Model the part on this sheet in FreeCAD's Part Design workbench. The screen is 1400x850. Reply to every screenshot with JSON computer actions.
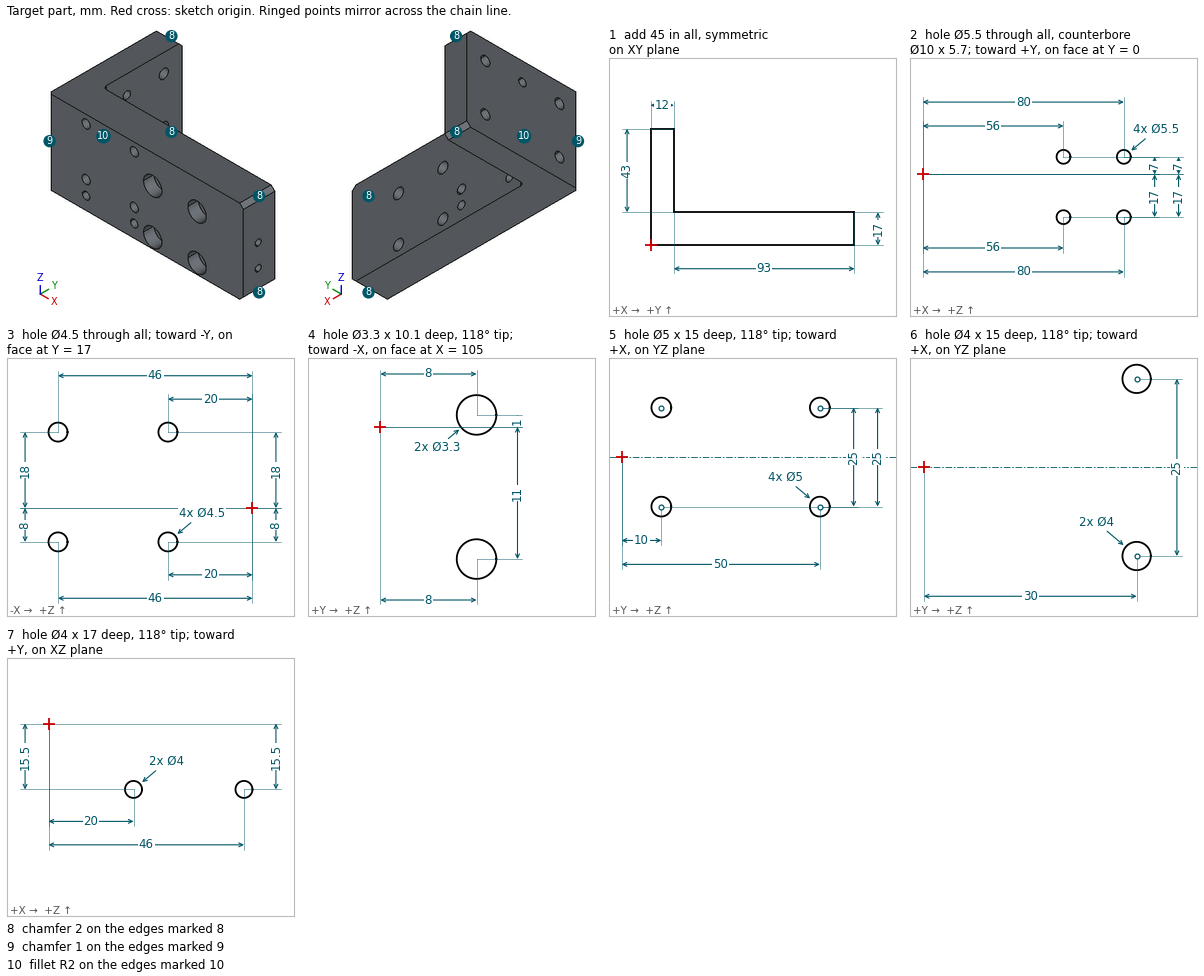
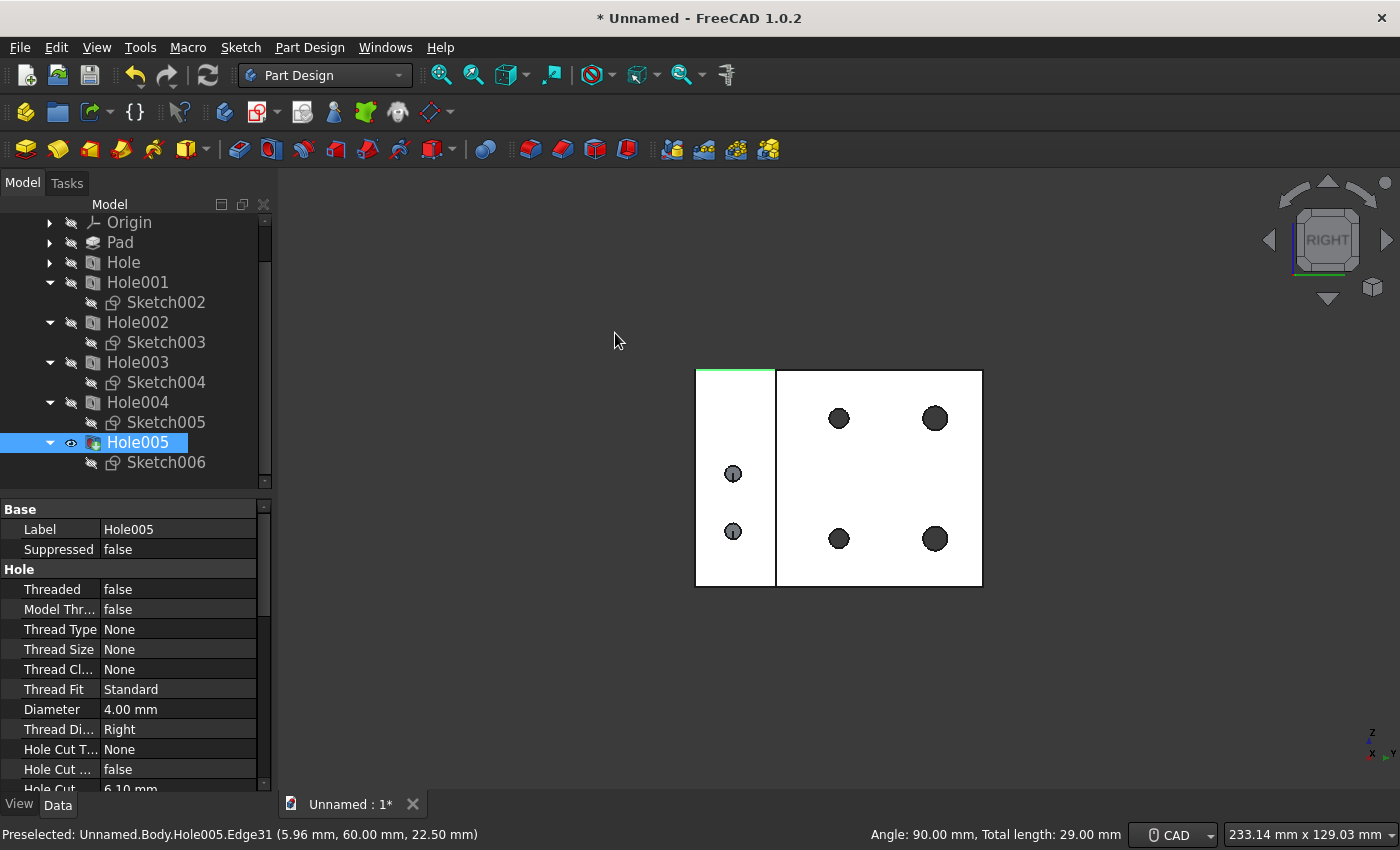
{"action": "left_click", "coordinate": [442, 76]}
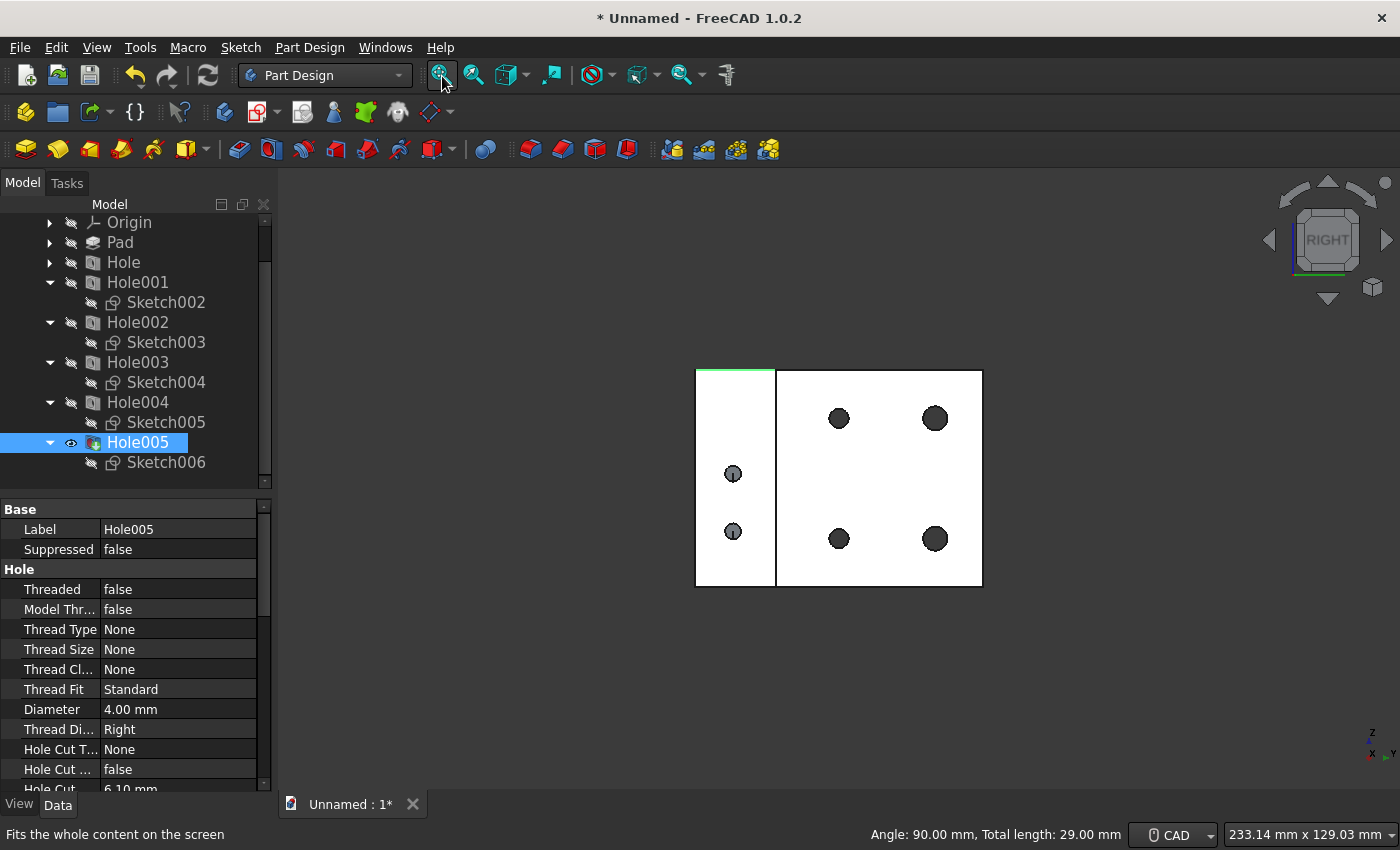
{"action": "left_click", "coordinate": [736, 586], "text": "ctrl"}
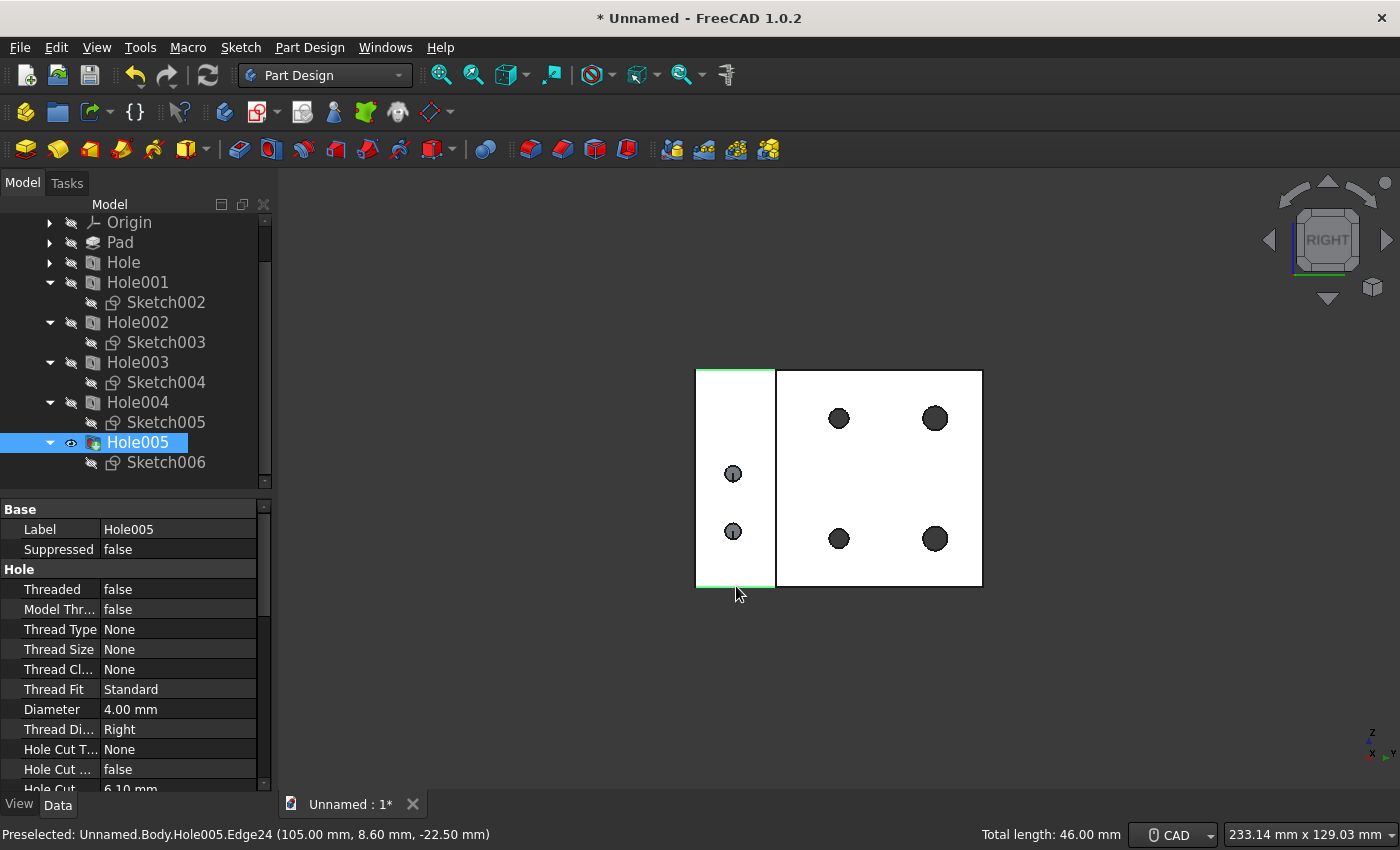
{"action": "key", "text": "5"}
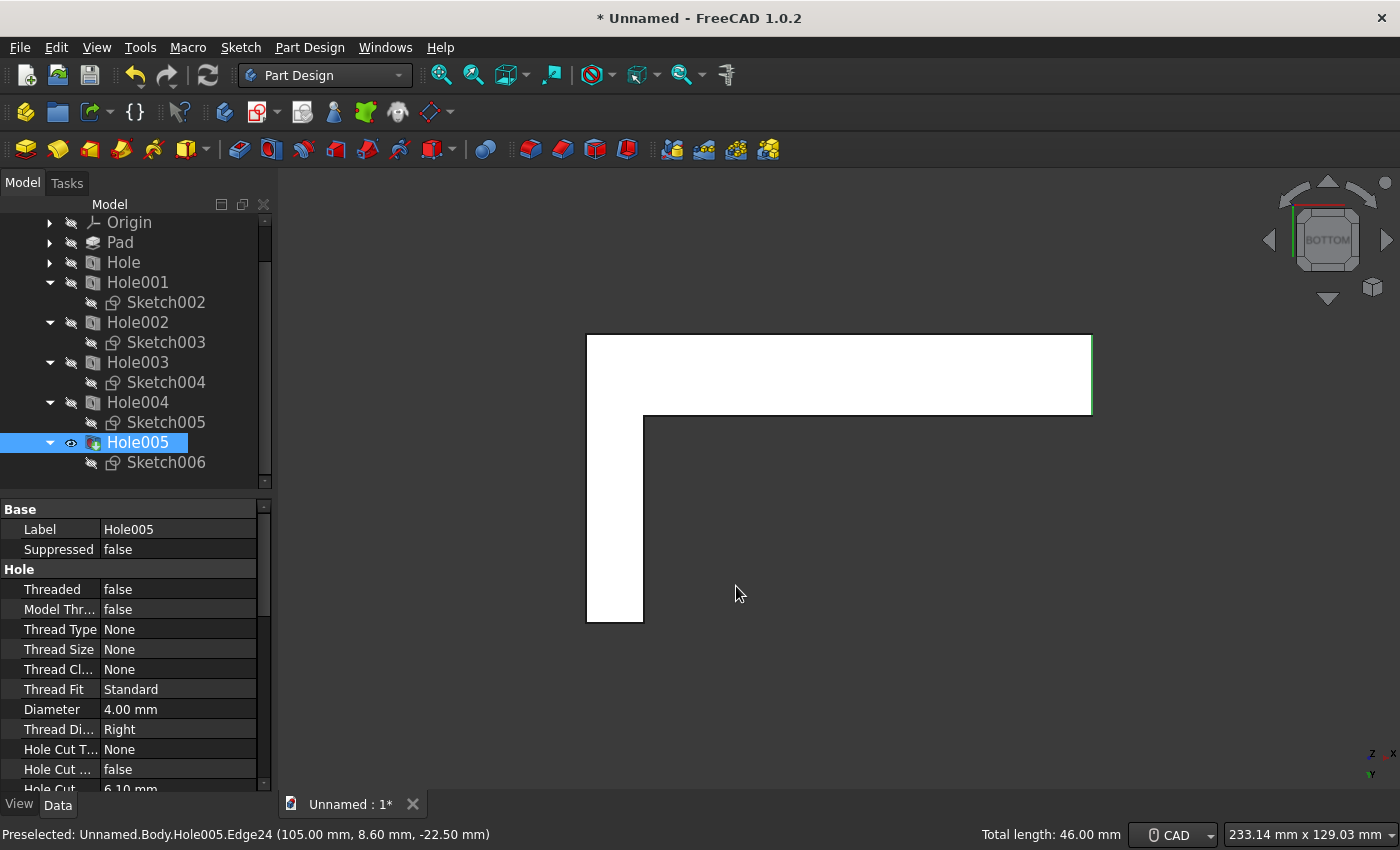
{"action": "left_click", "coordinate": [615, 622], "text": "ctrl"}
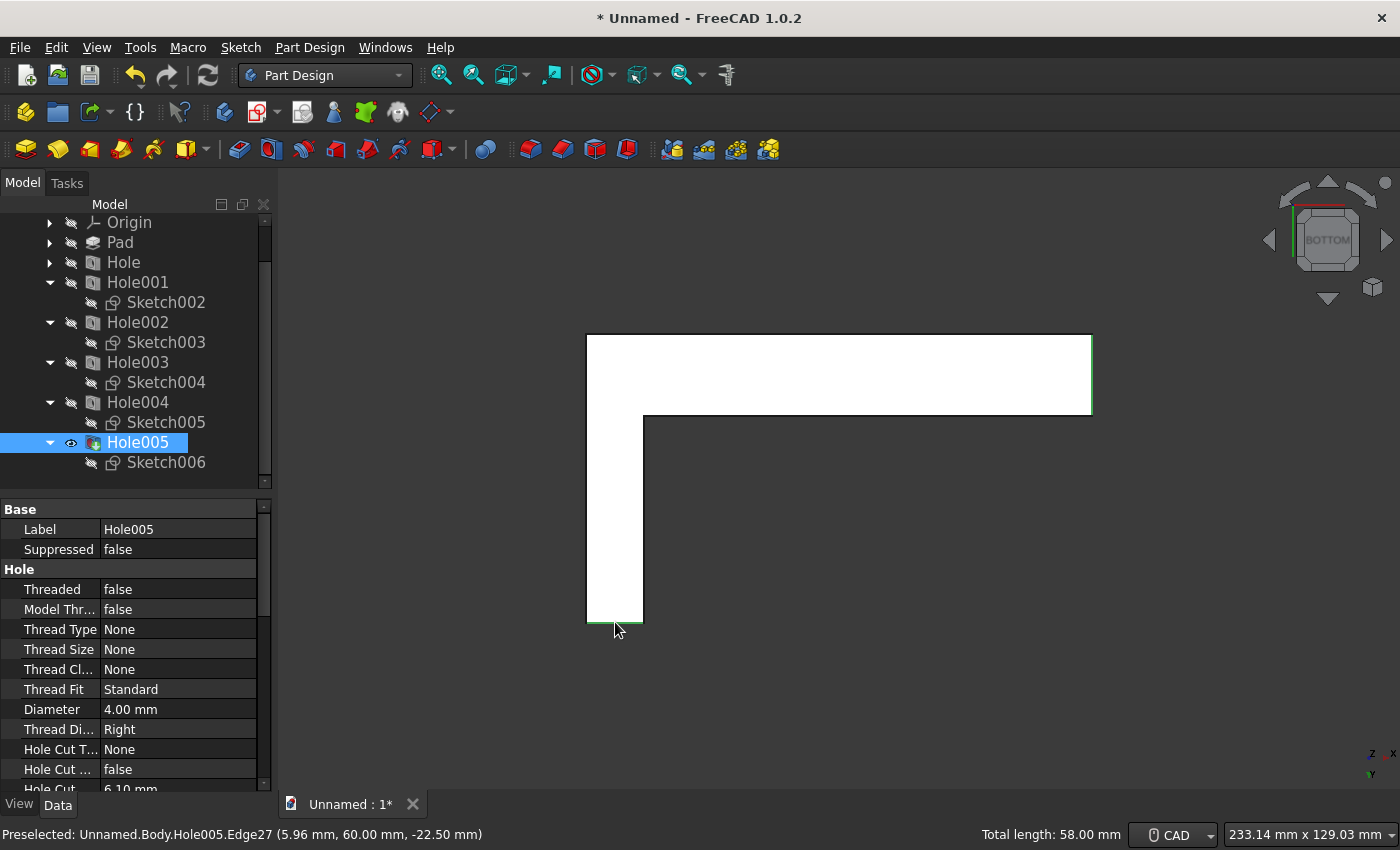
{"action": "left_click", "coordinate": [564, 150]}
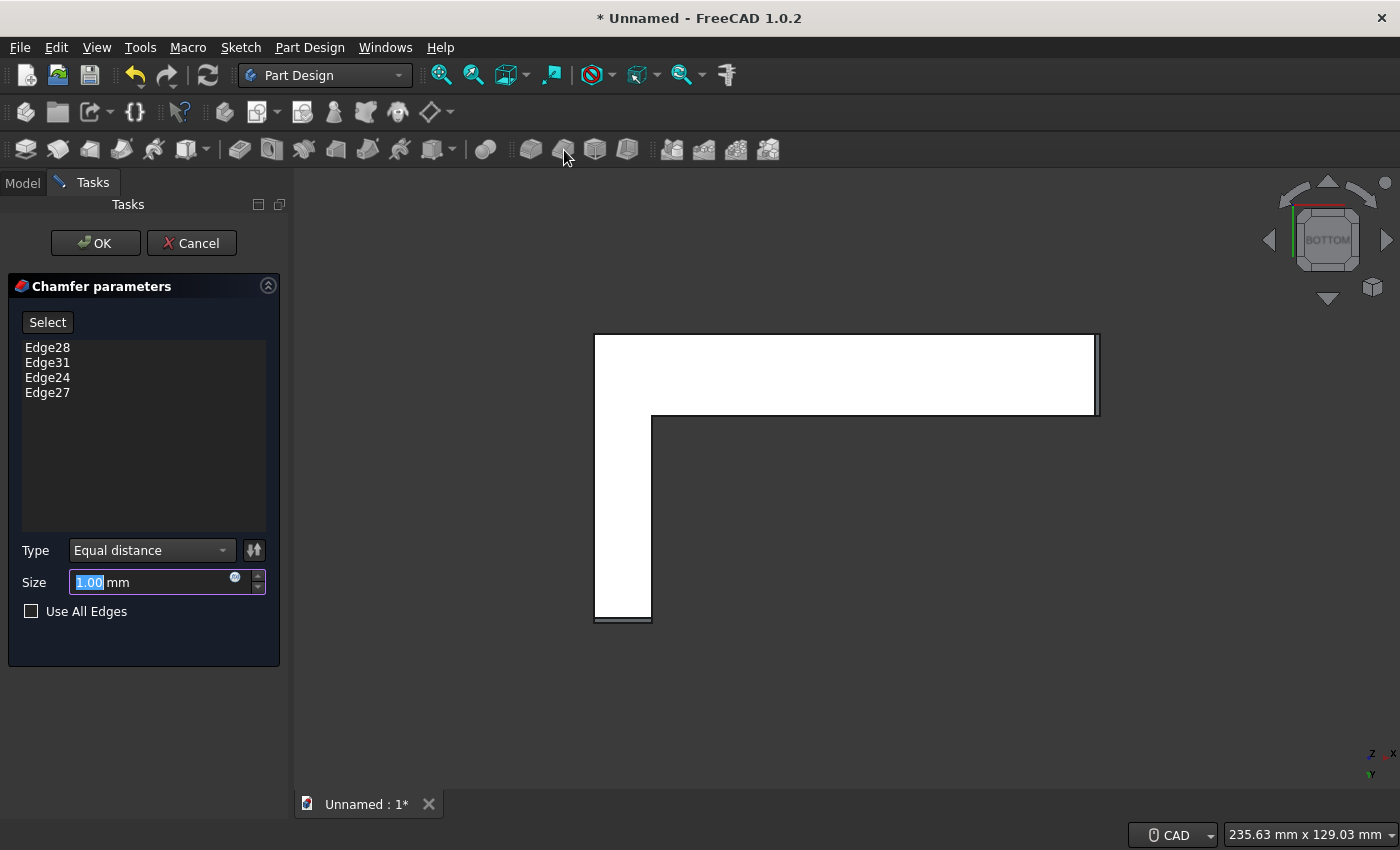
{"action": "type", "text": "2"}
{"action": "key", "text": "Tab"}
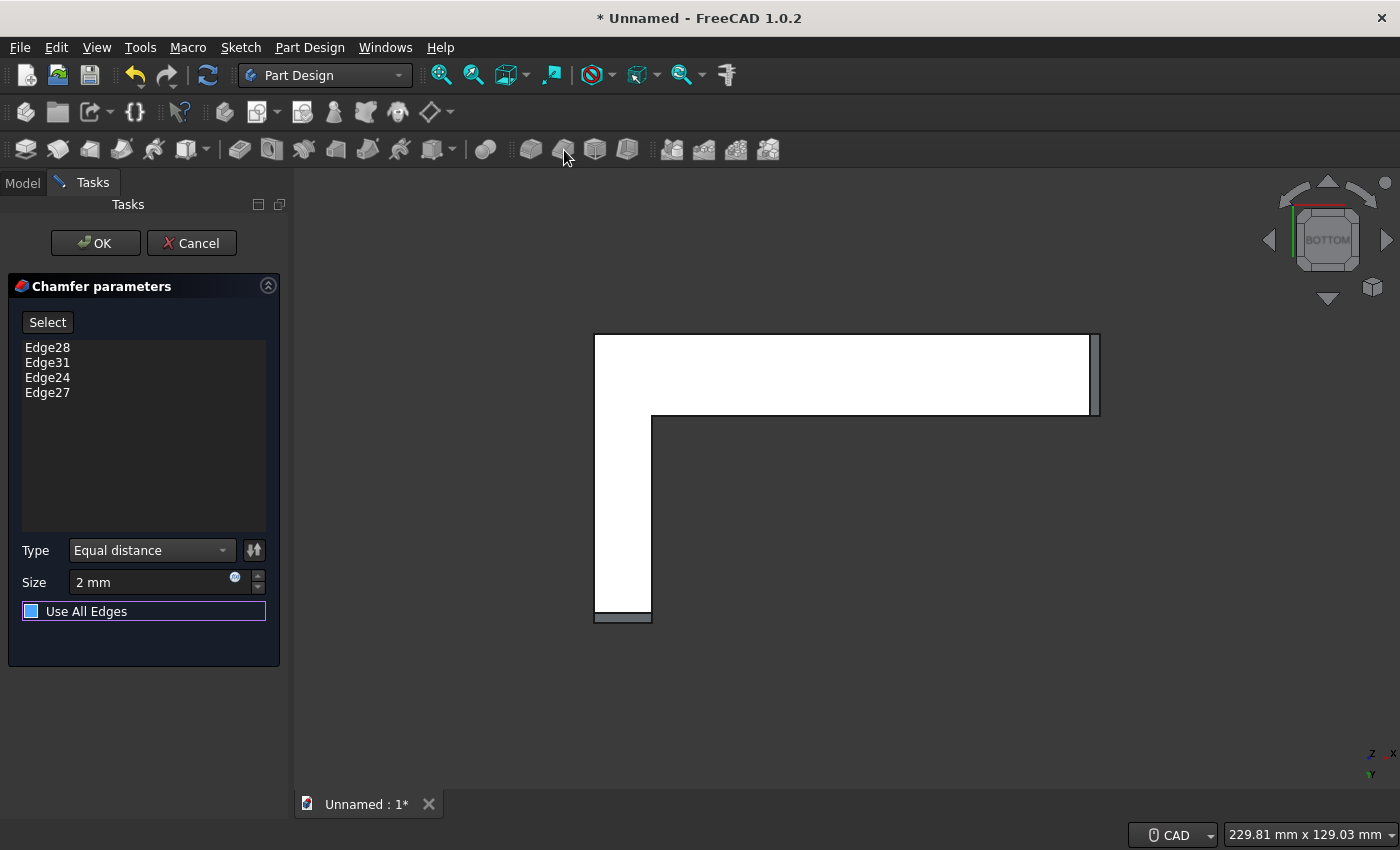
{"action": "left_click", "coordinate": [96, 243]}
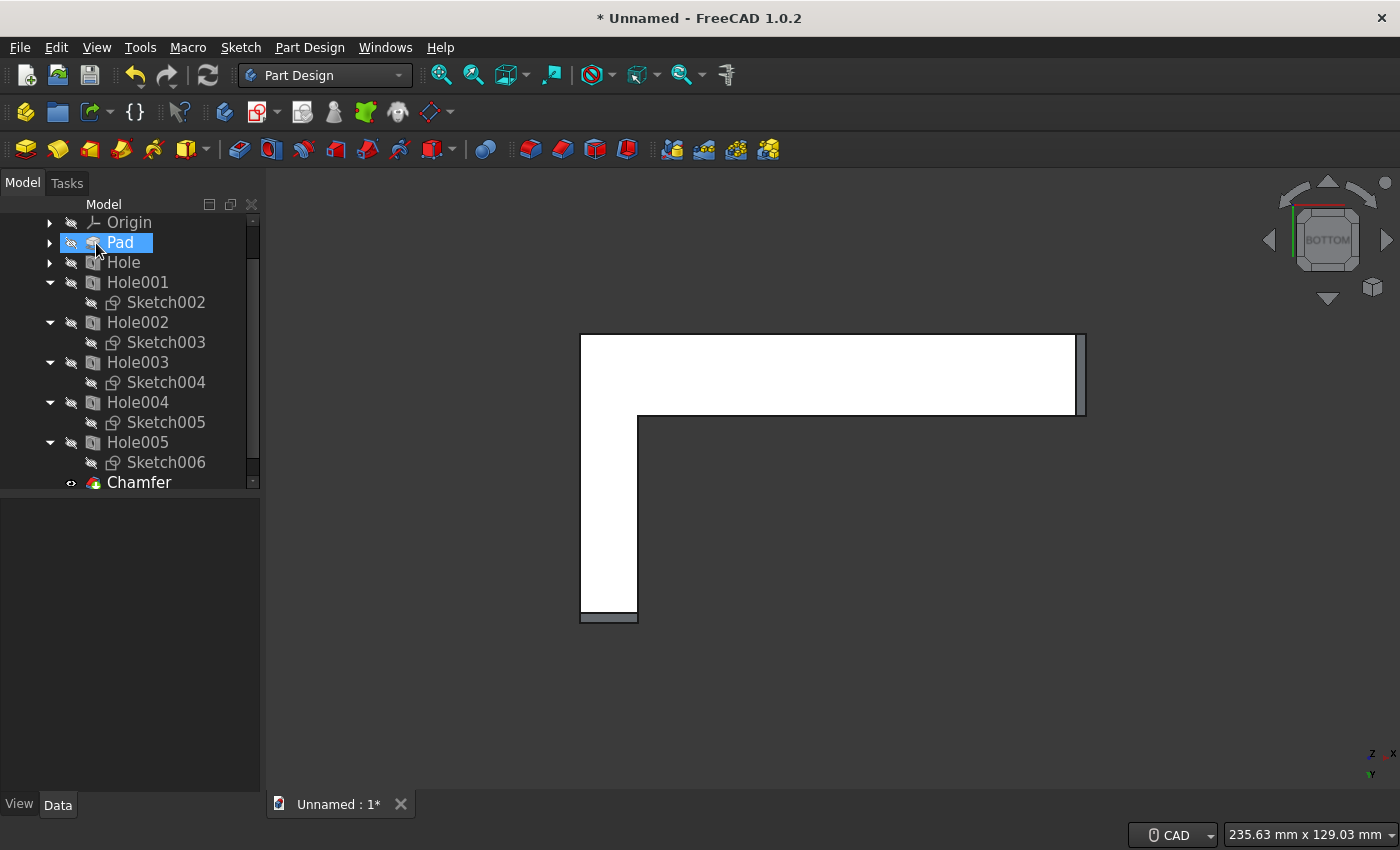
{"action": "key", "text": "0"}